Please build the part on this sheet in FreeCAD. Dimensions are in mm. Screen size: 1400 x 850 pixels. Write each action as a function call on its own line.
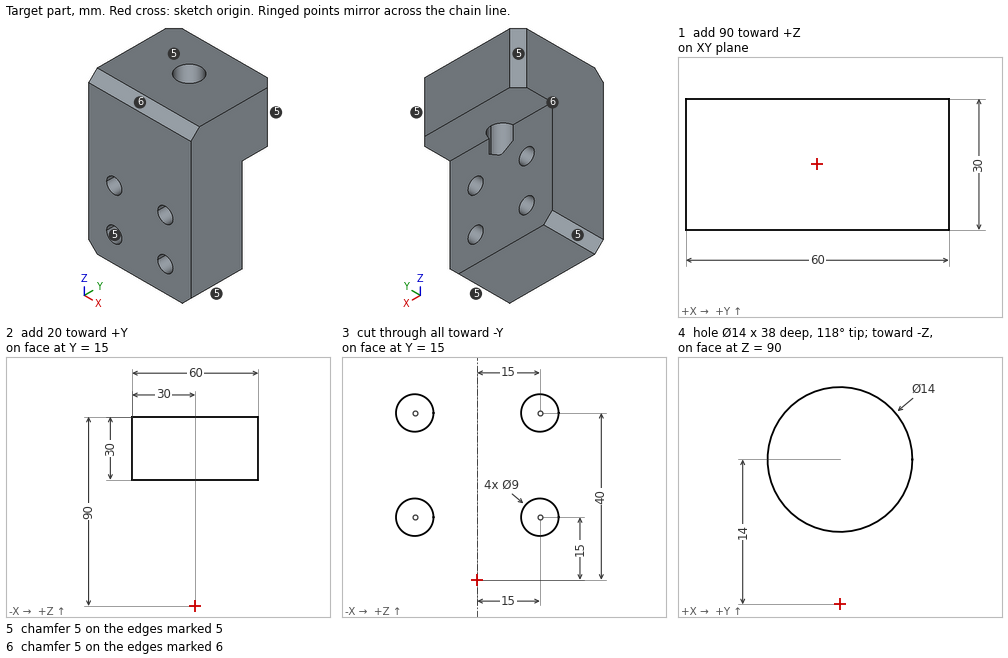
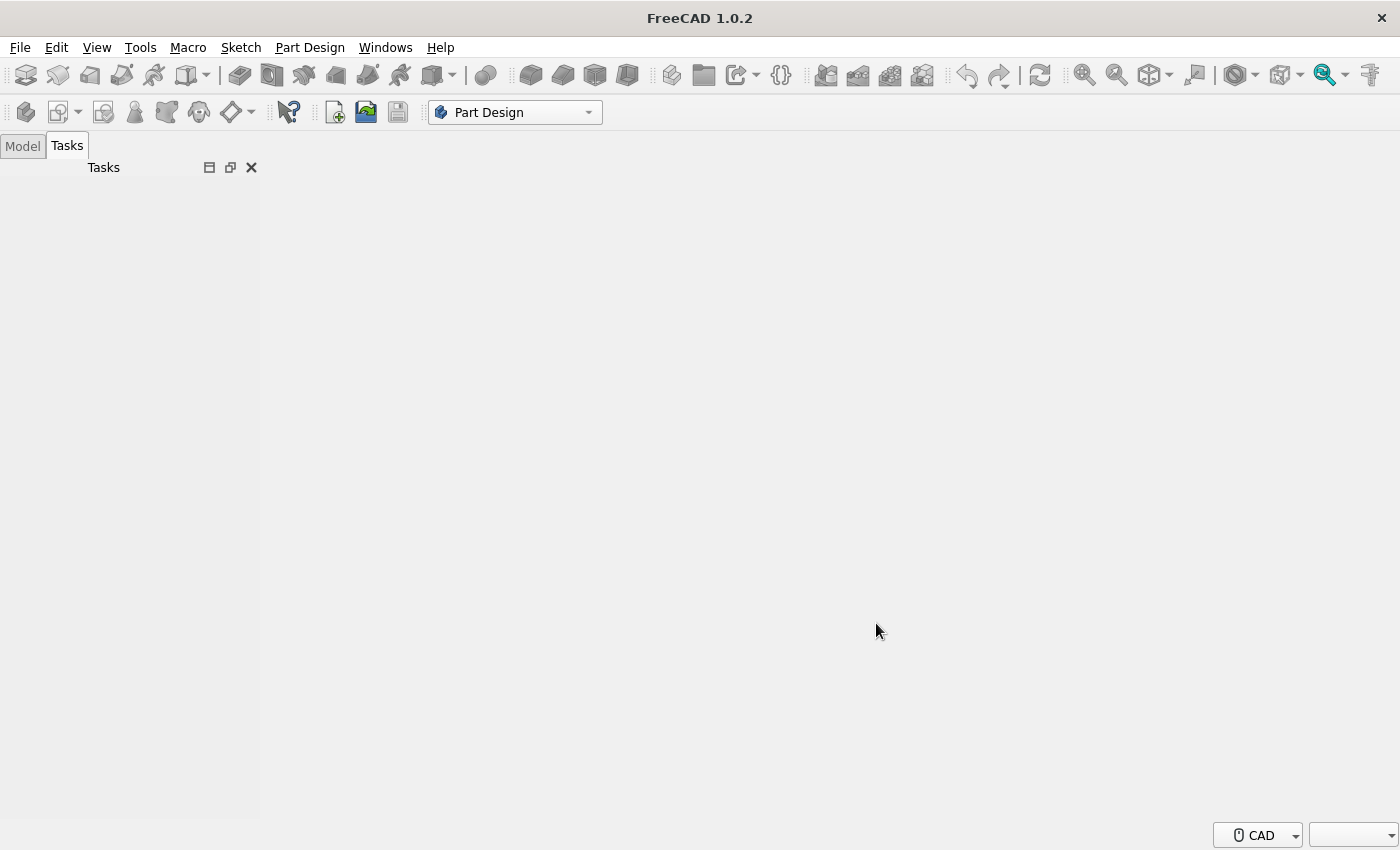
click(334, 112)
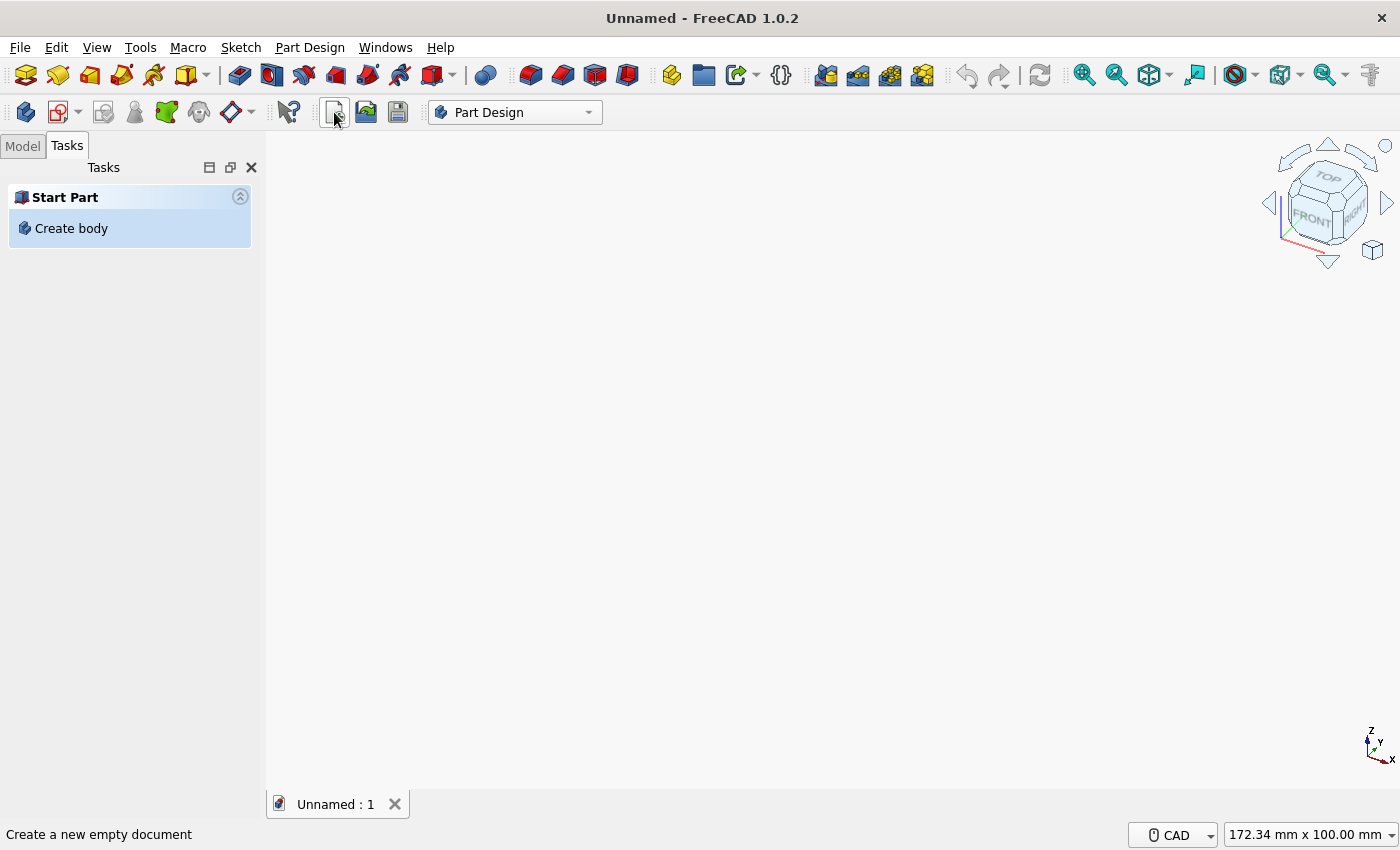
click(58, 112)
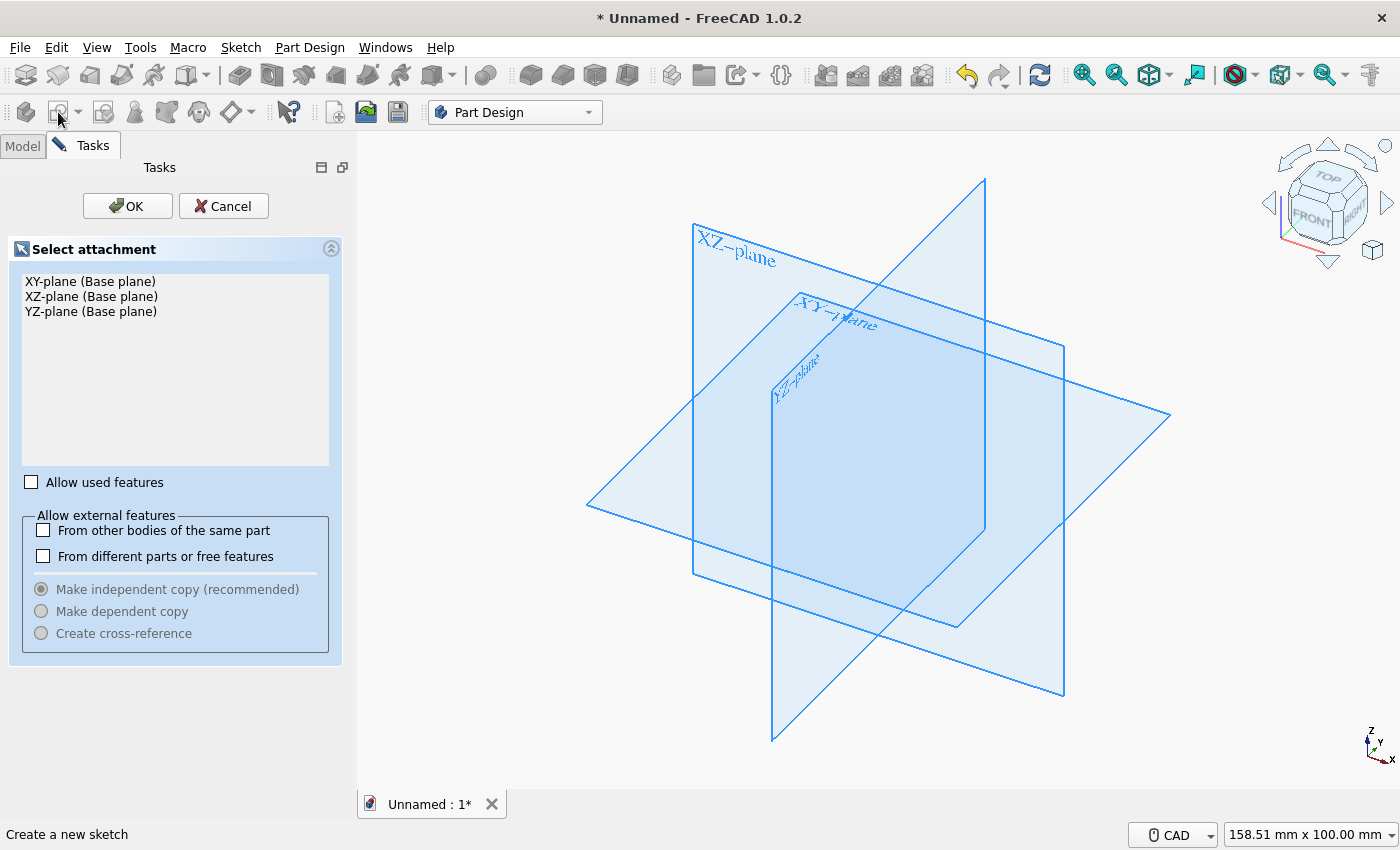
click(82, 282)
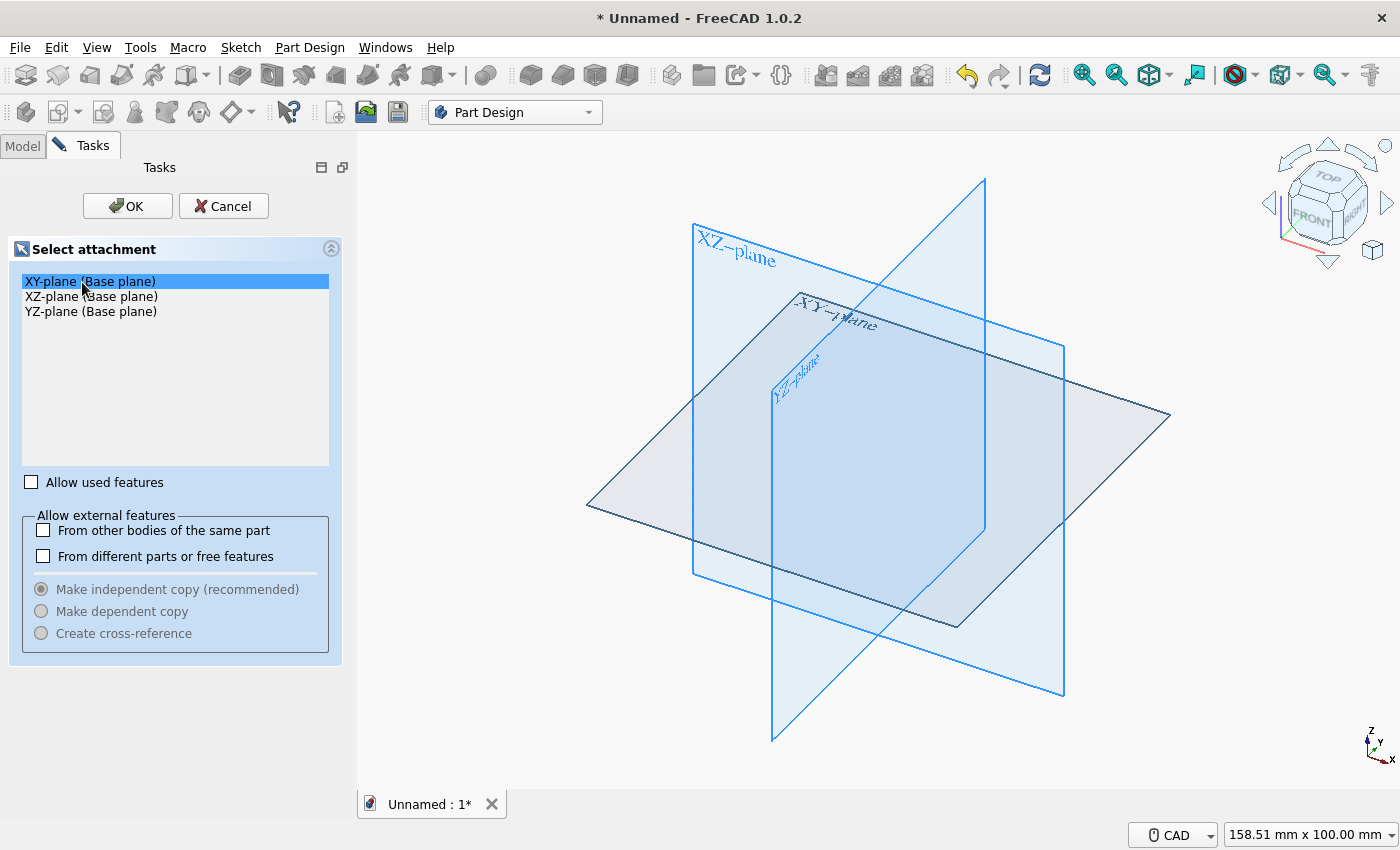
click(128, 206)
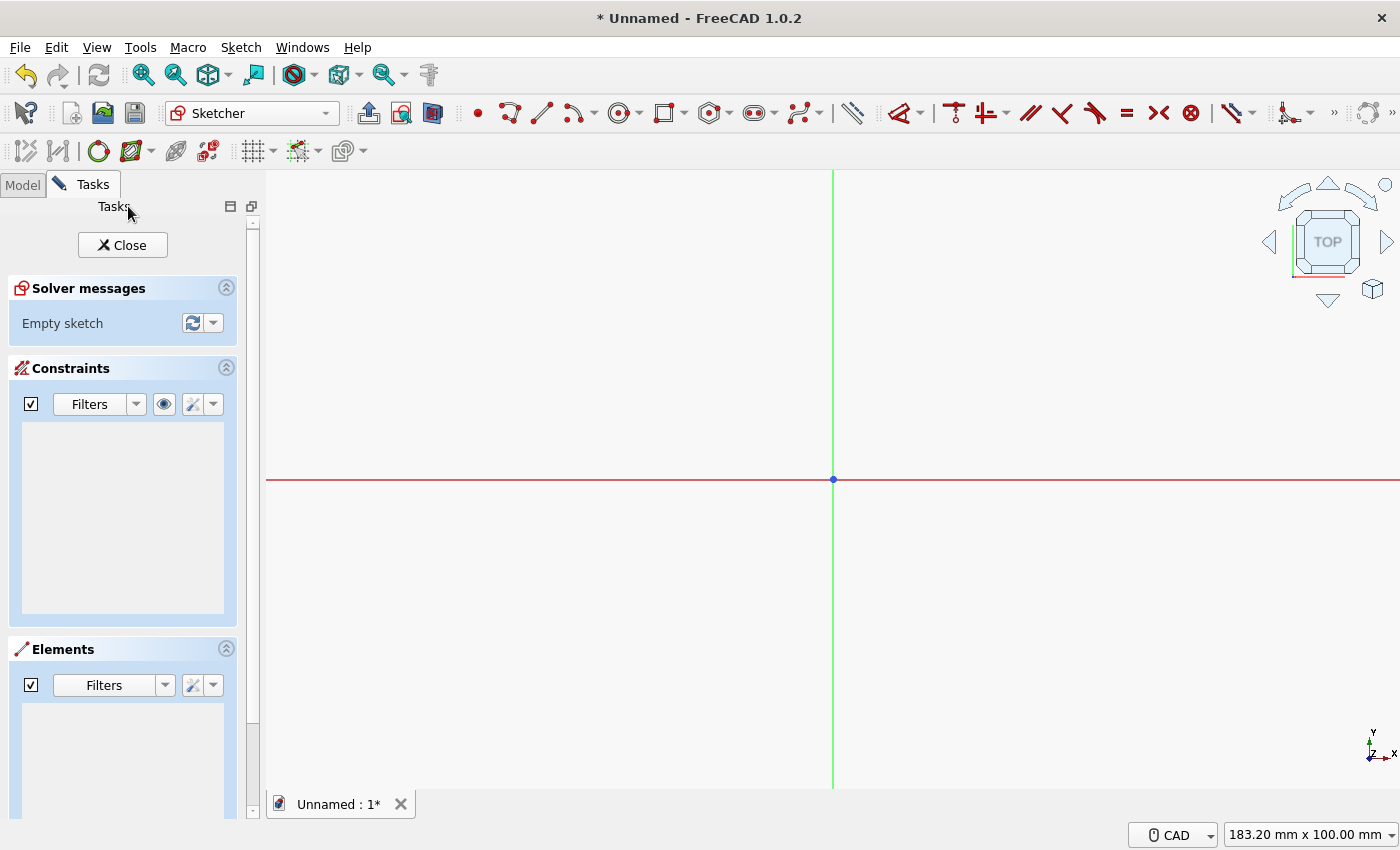
scroll(916, 480, up, 3)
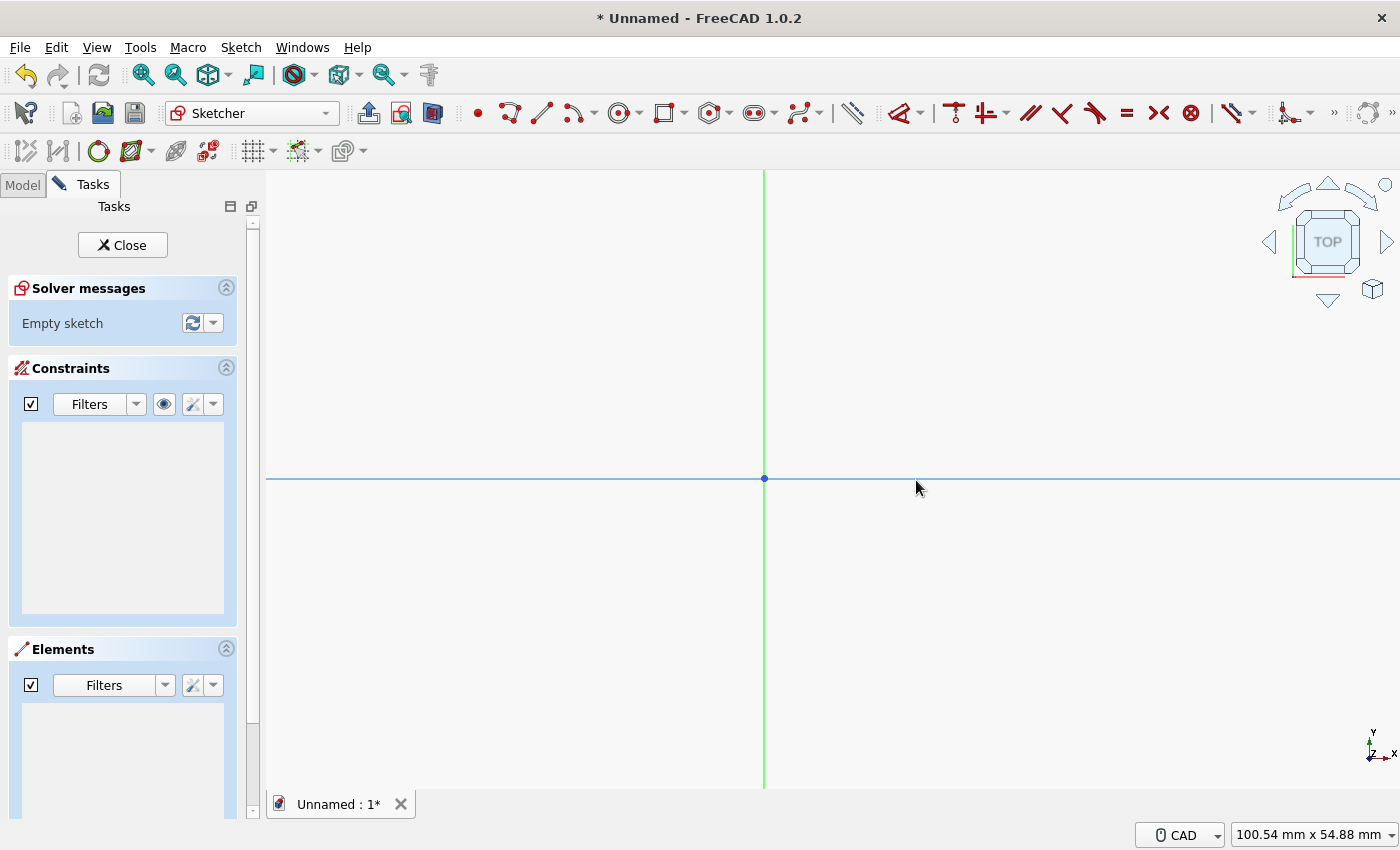
key(g)
key(v)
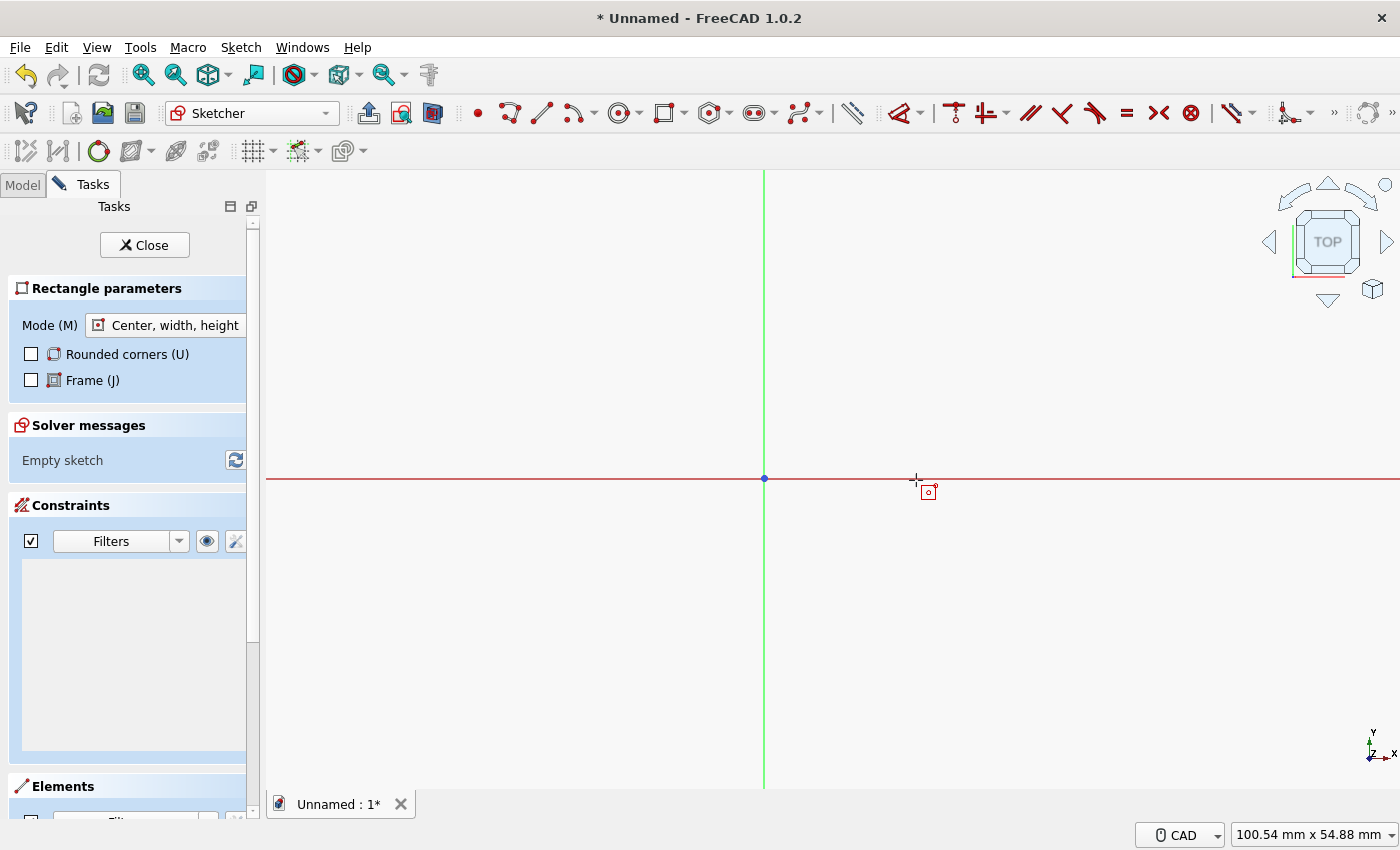
click(764, 479)
click(1103, 309)
key(Escape)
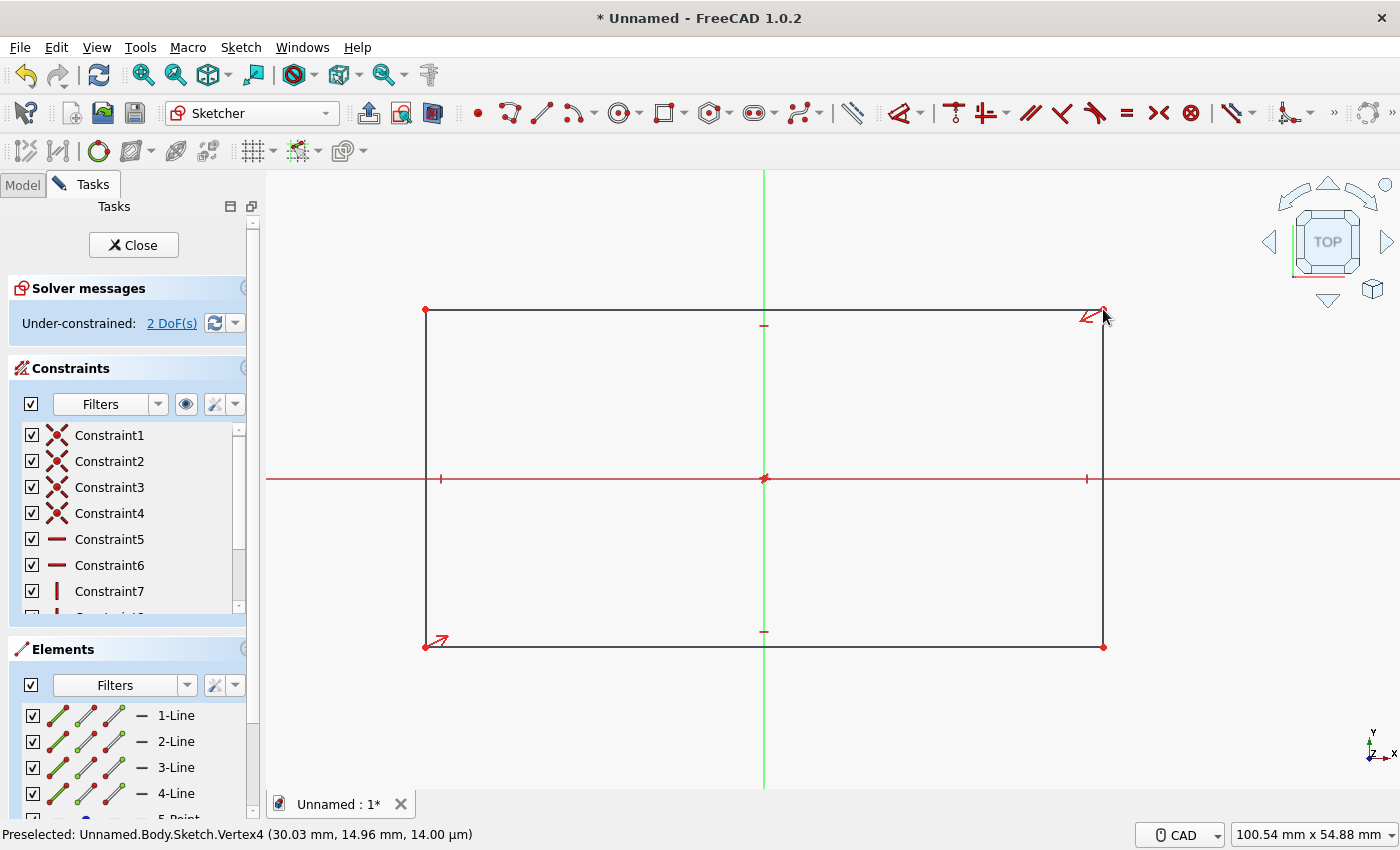
click(629, 647)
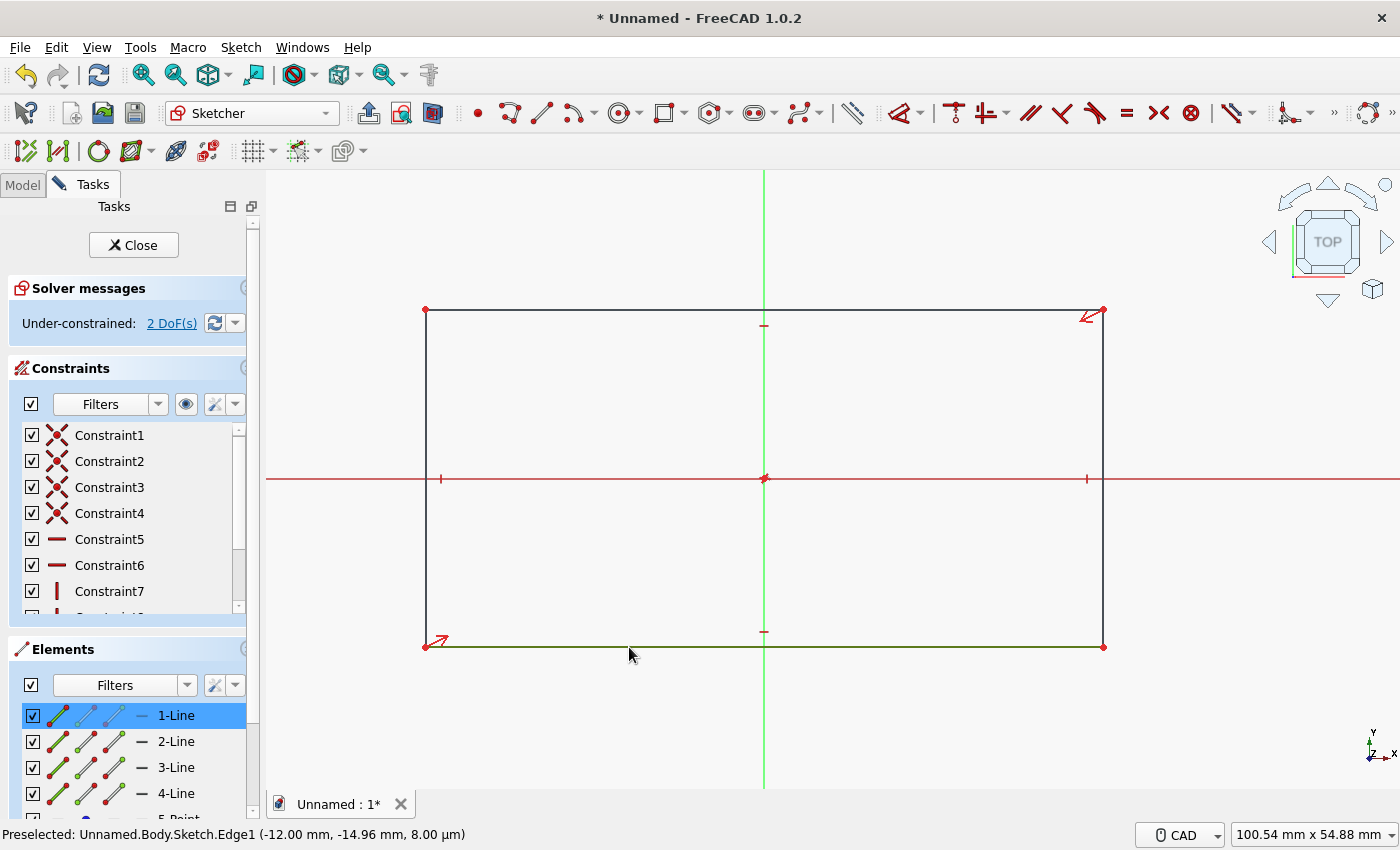
click(922, 114)